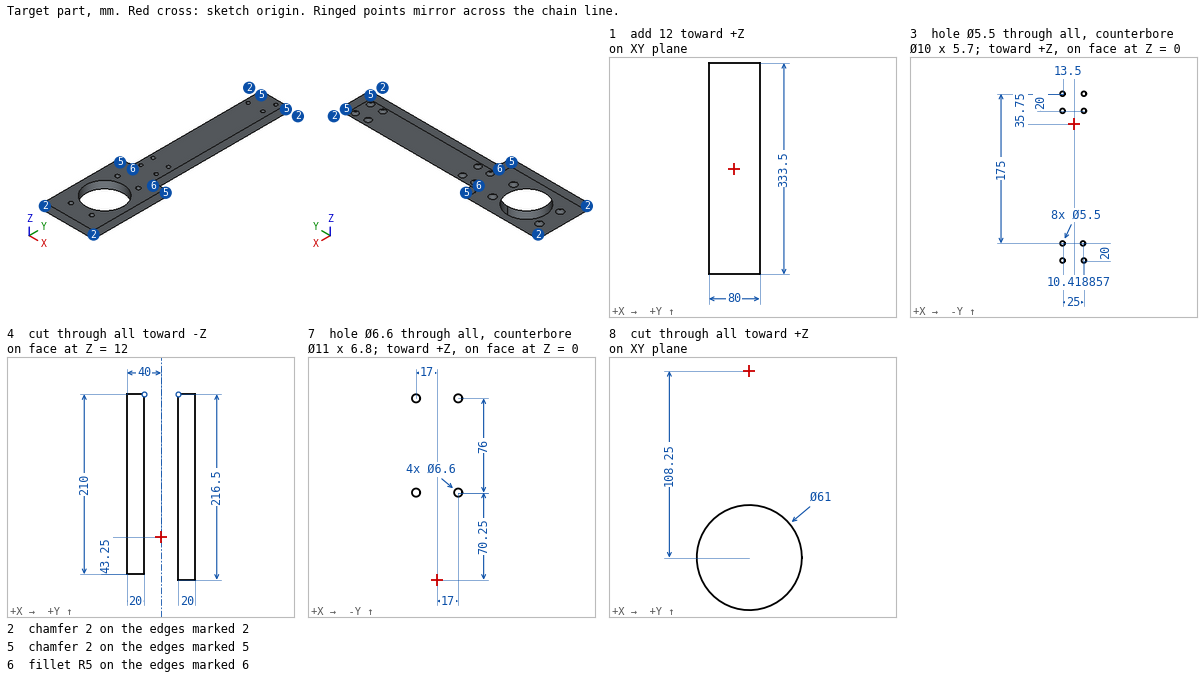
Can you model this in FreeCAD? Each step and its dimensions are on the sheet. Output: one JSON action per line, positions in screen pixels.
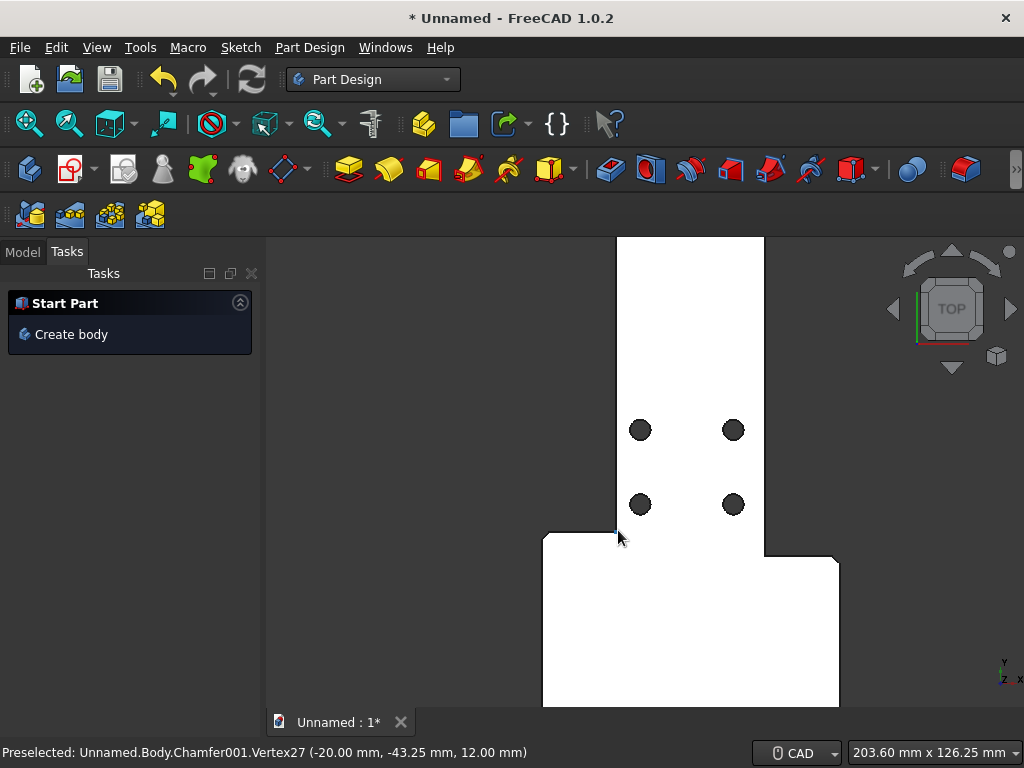
{"action": "key", "text": "v f"}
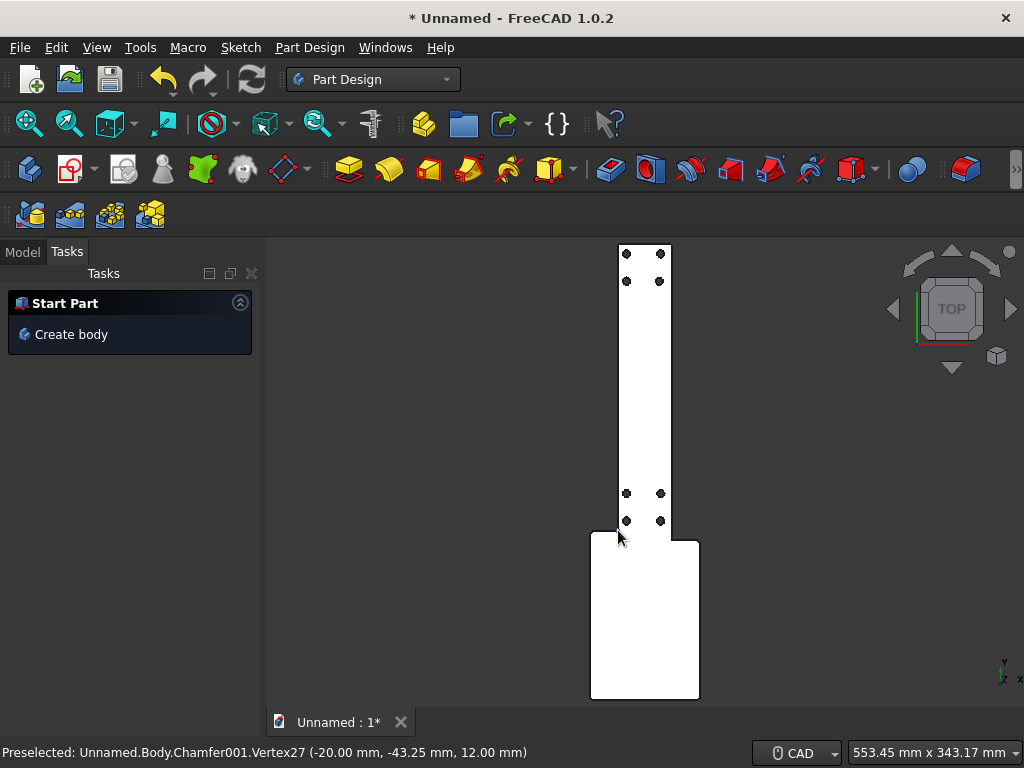
{"action": "key", "text": "1"}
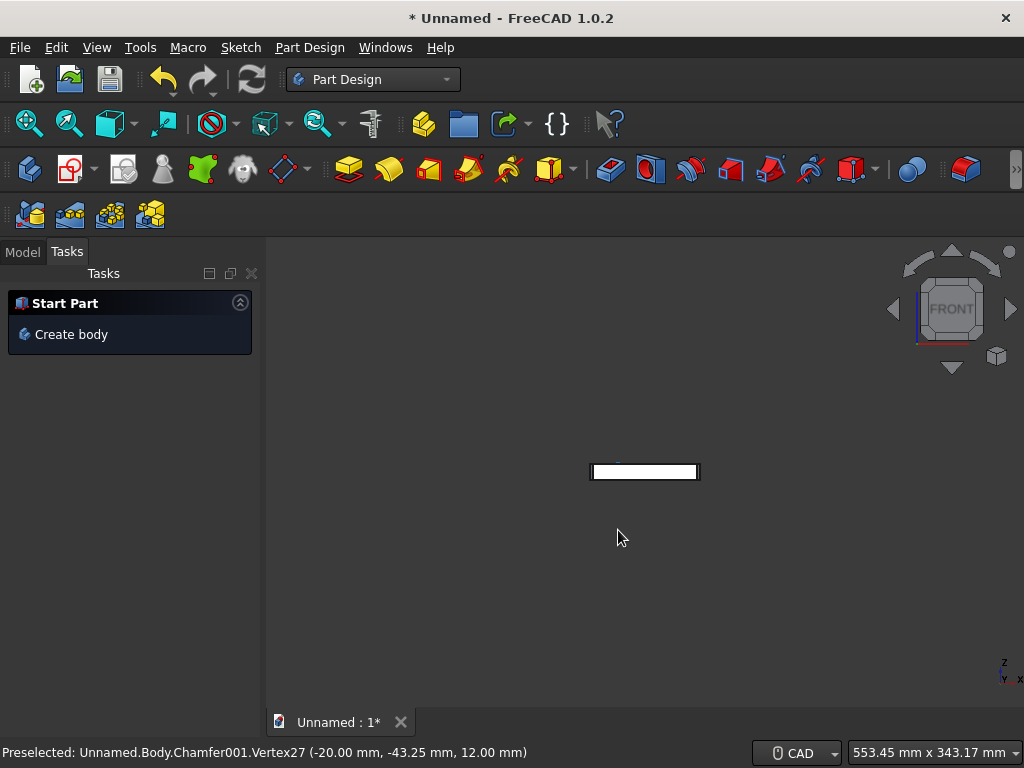
{"action": "key", "text": "v f"}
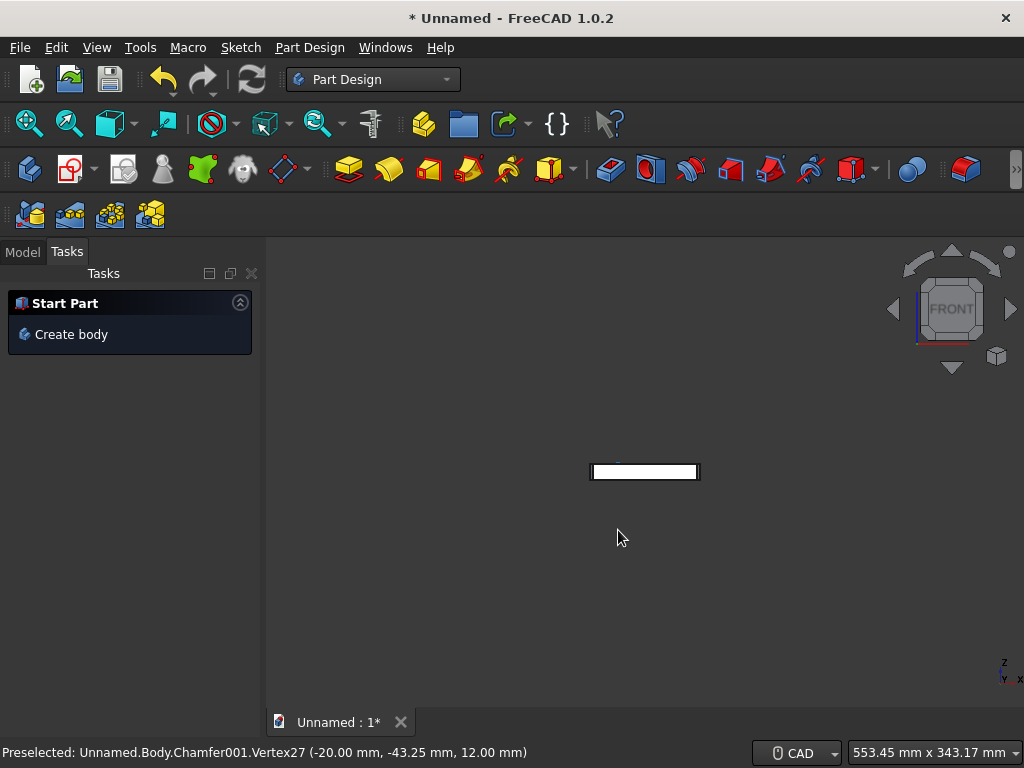
{"action": "scroll", "coordinate": [618, 471], "scroll_direction": "up", "scroll_amount": 5}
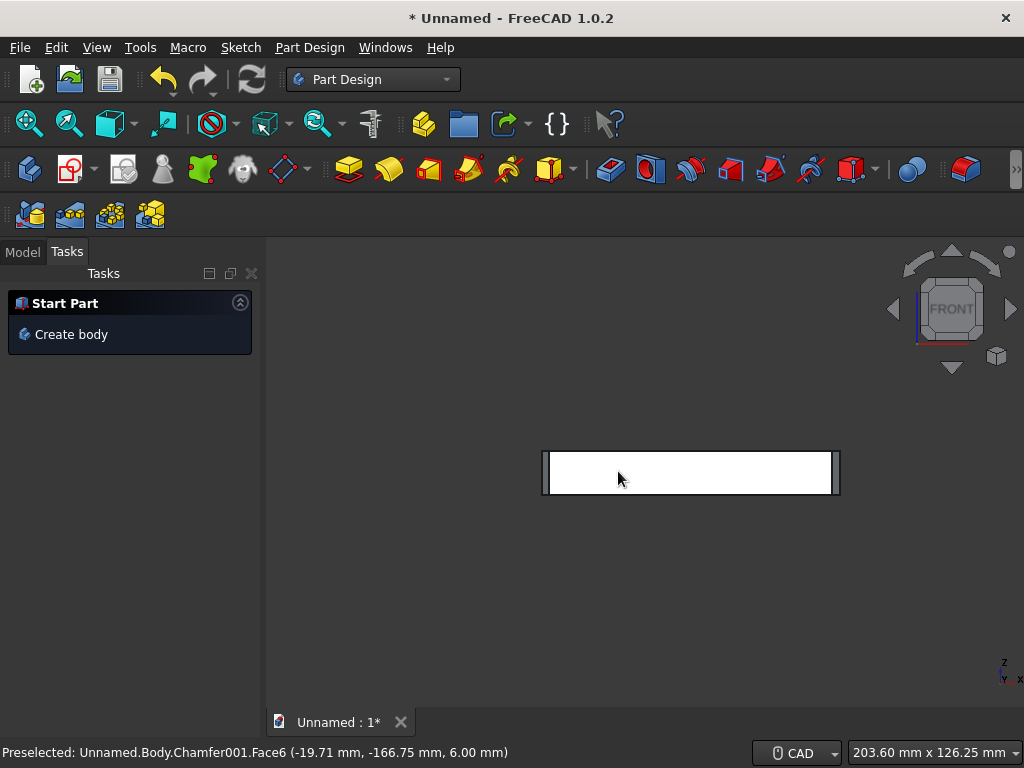
{"action": "key", "text": "v f"}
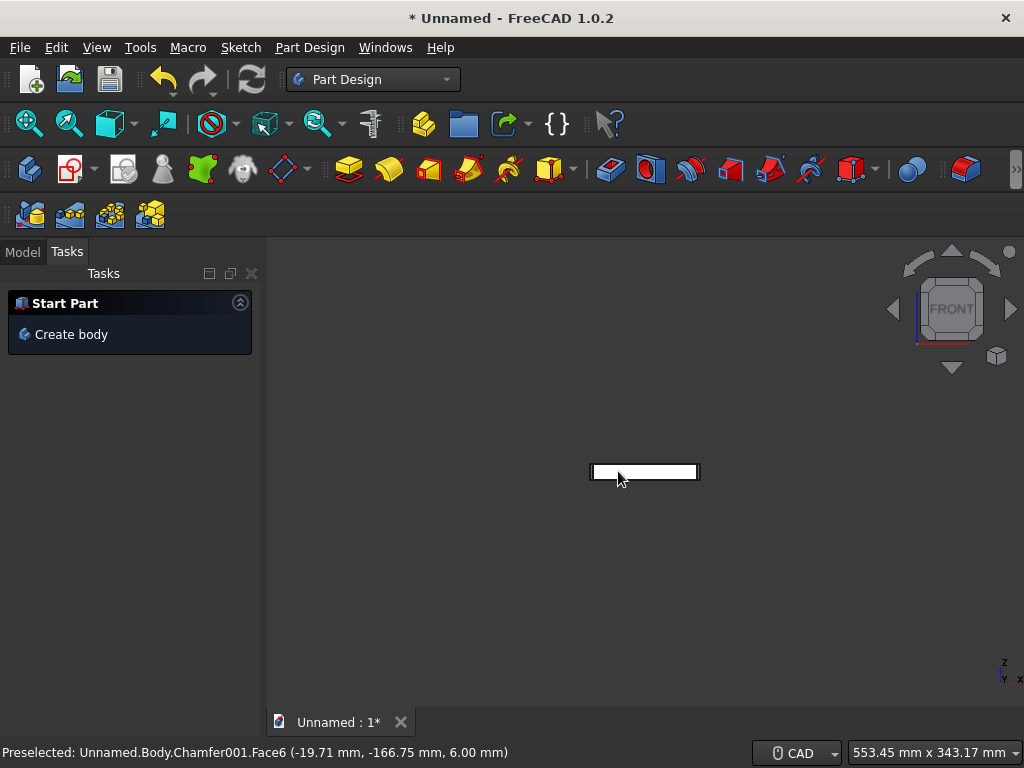
{"action": "key", "text": "3"}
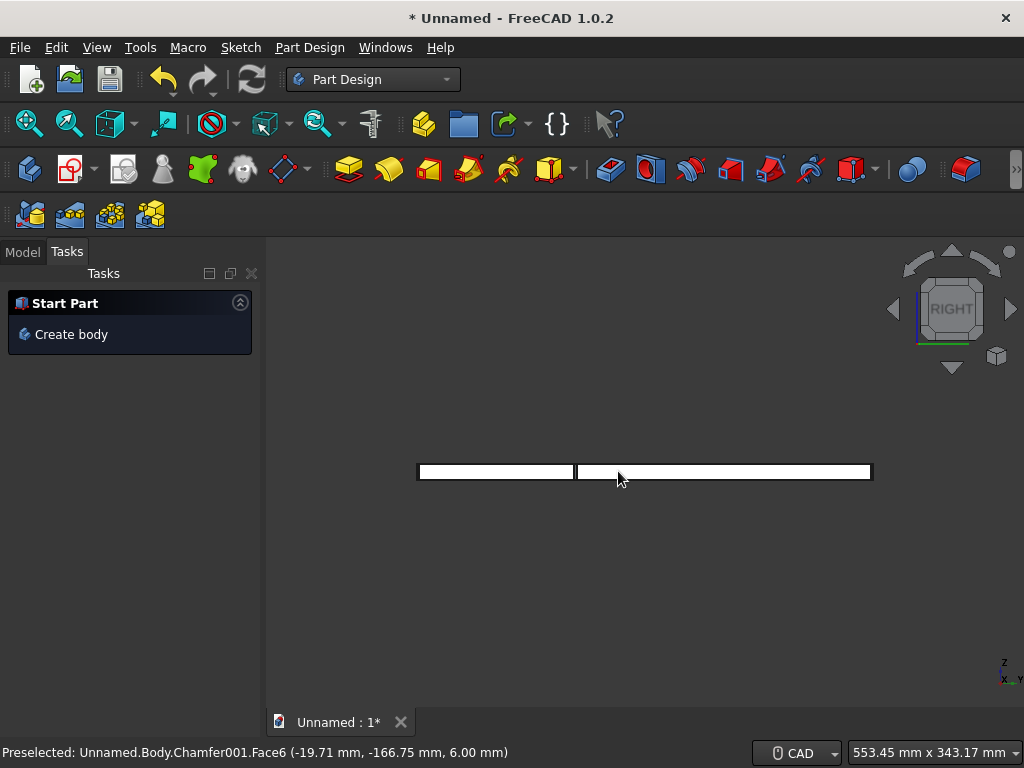
{"action": "scroll", "coordinate": [586, 471], "scroll_direction": "up", "scroll_amount": 5}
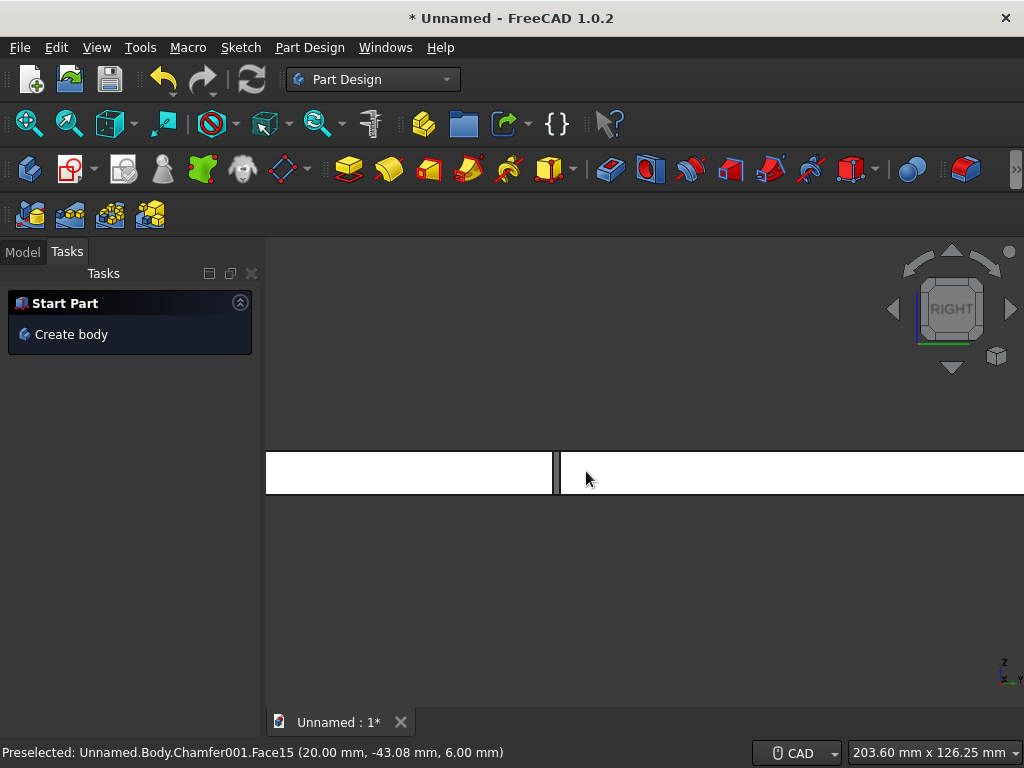
{"action": "key", "text": "v f"}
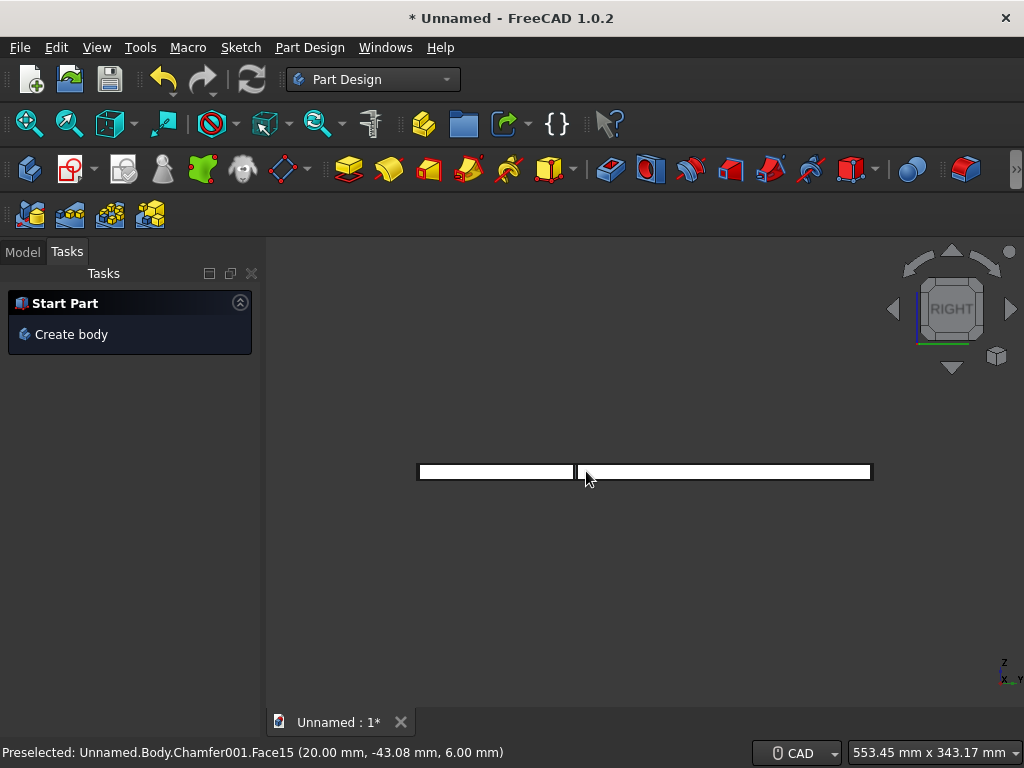
{"action": "key", "text": "5"}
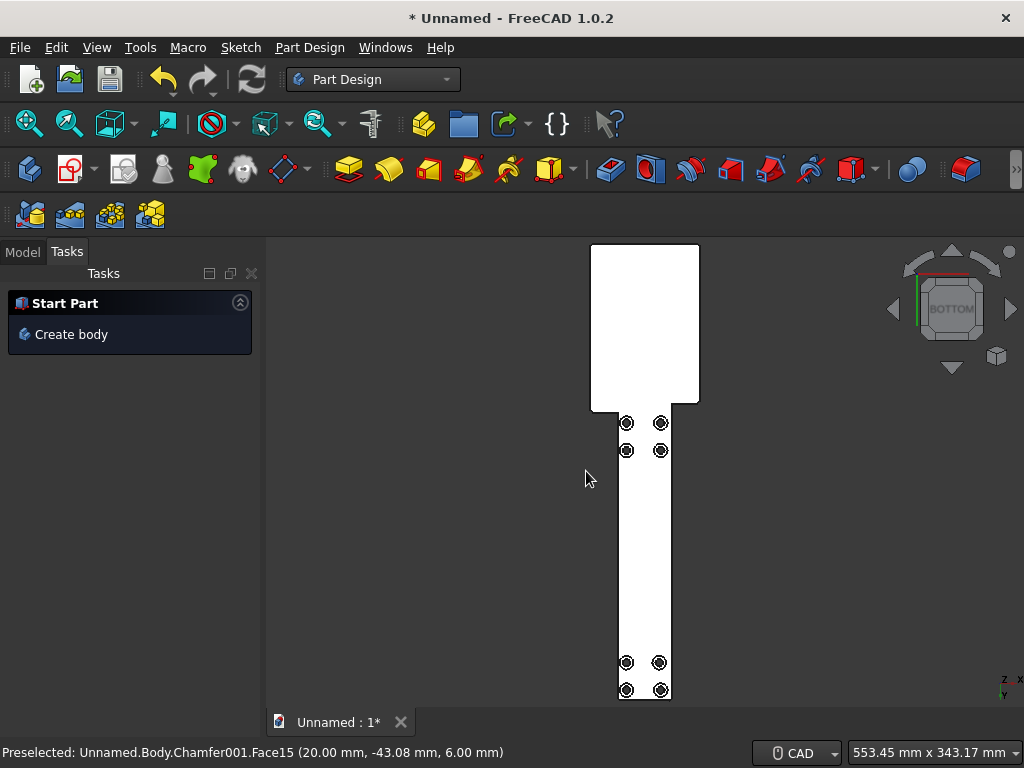
{"action": "scroll", "coordinate": [618, 412], "scroll_direction": "up", "scroll_amount": 5}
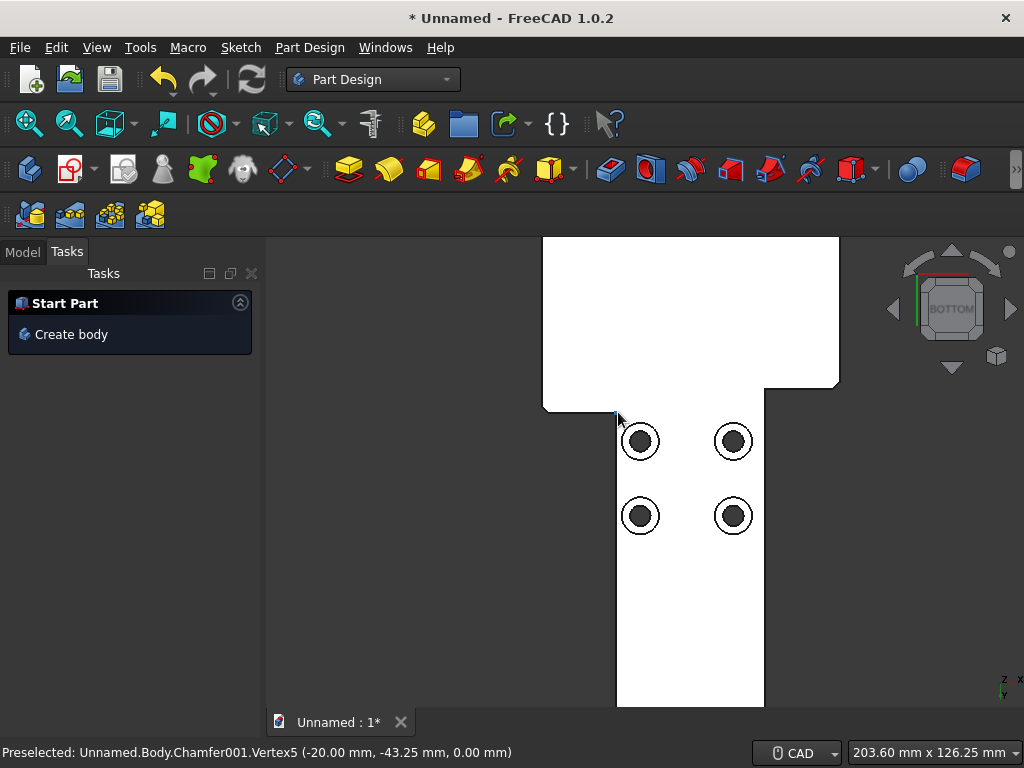
{"action": "key", "text": "v f"}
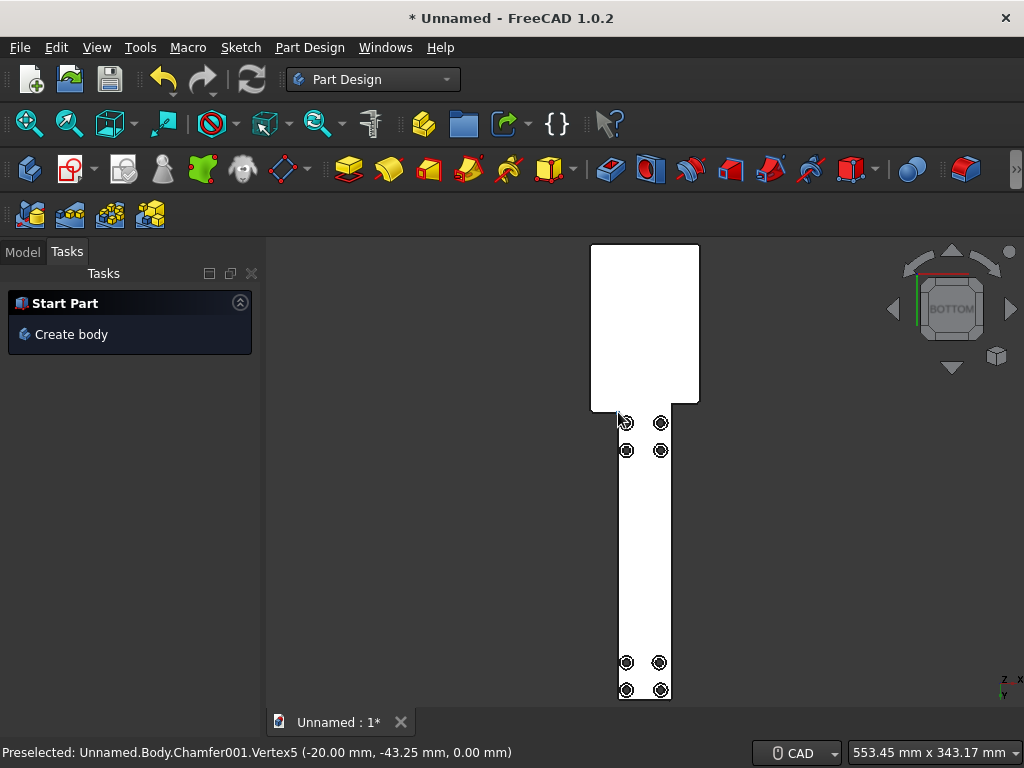
{"action": "key", "text": "4"}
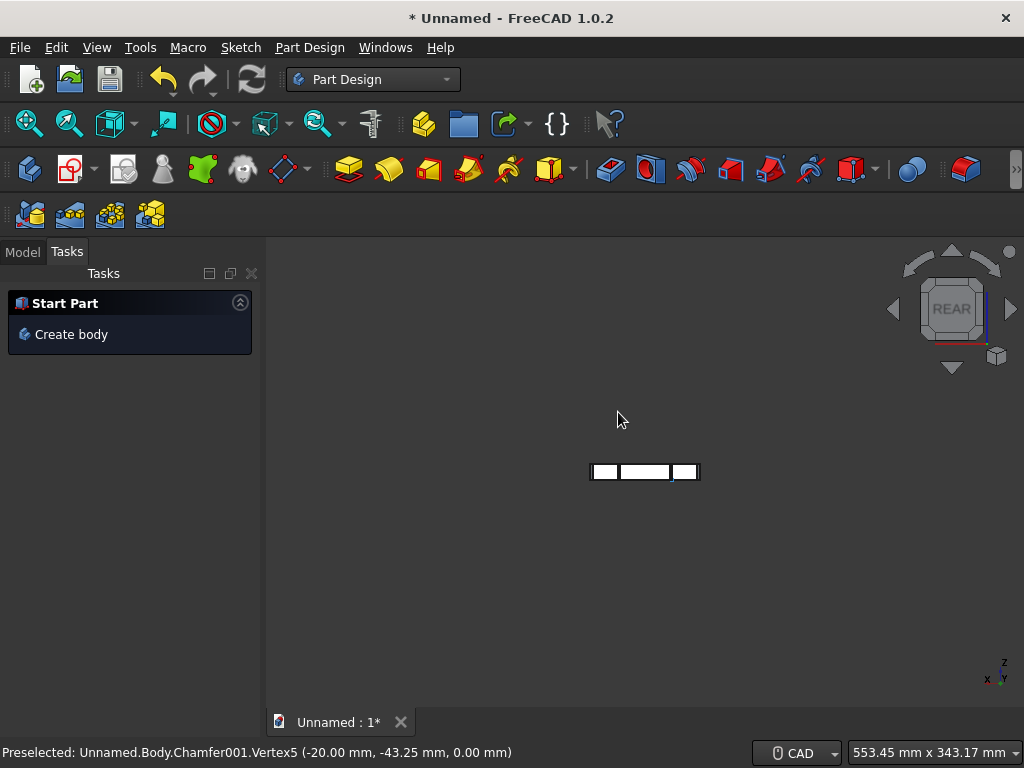
{"action": "left_click", "coordinate": [30, 124]}